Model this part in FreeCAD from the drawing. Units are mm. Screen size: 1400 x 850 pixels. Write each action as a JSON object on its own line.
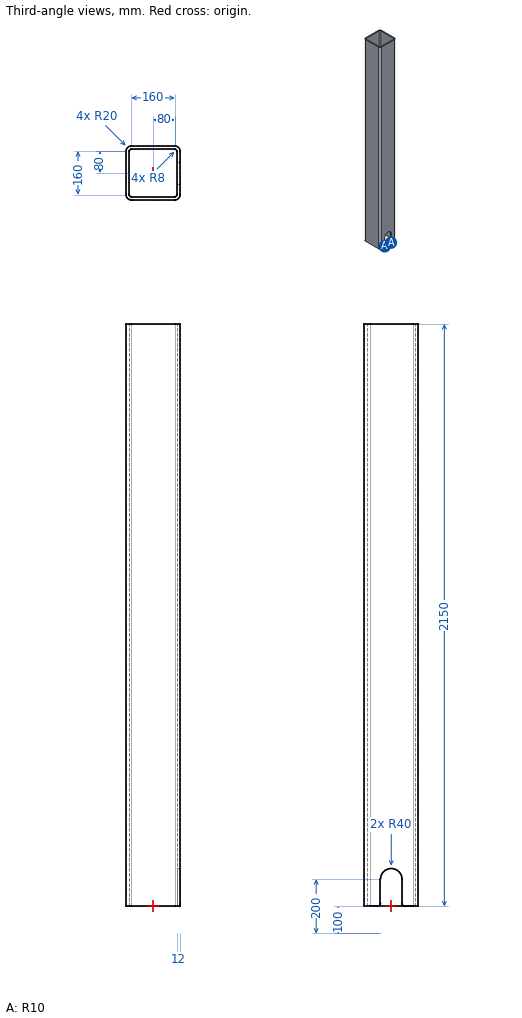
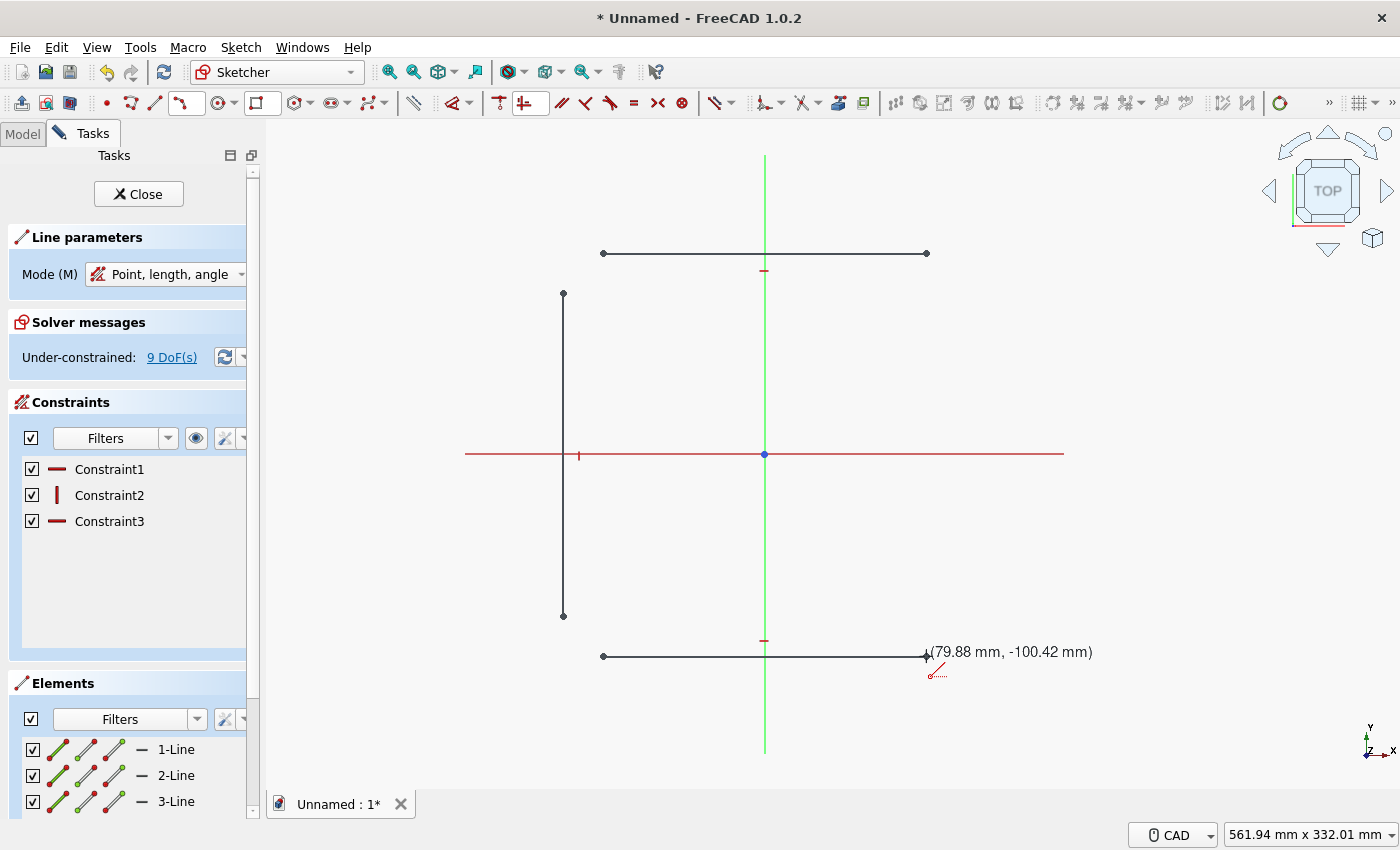
{"action": "left_click", "coordinate": [967, 616]}
{"action": "left_click", "coordinate": [967, 293]}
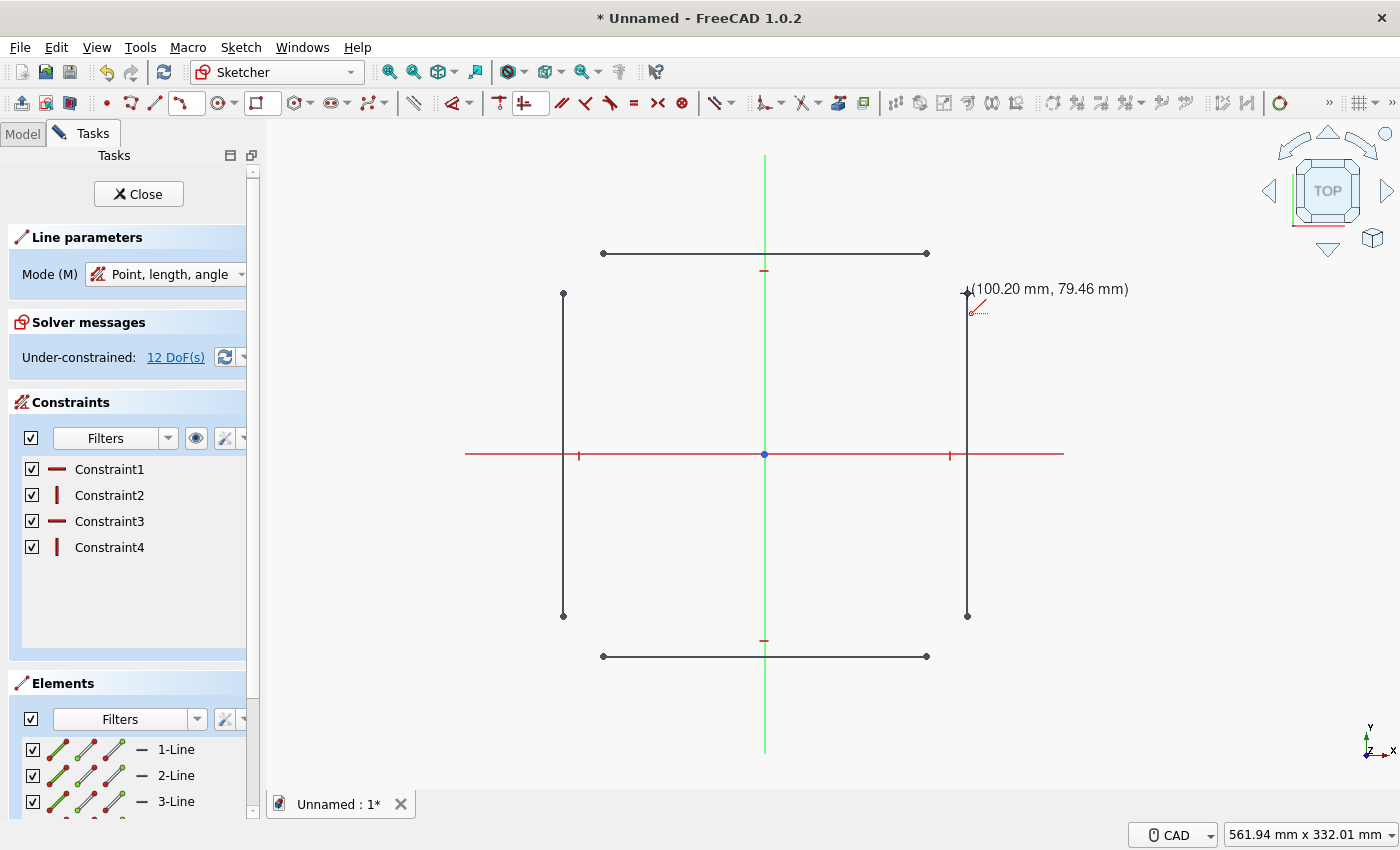
{"action": "left_click", "coordinate": [180, 104]}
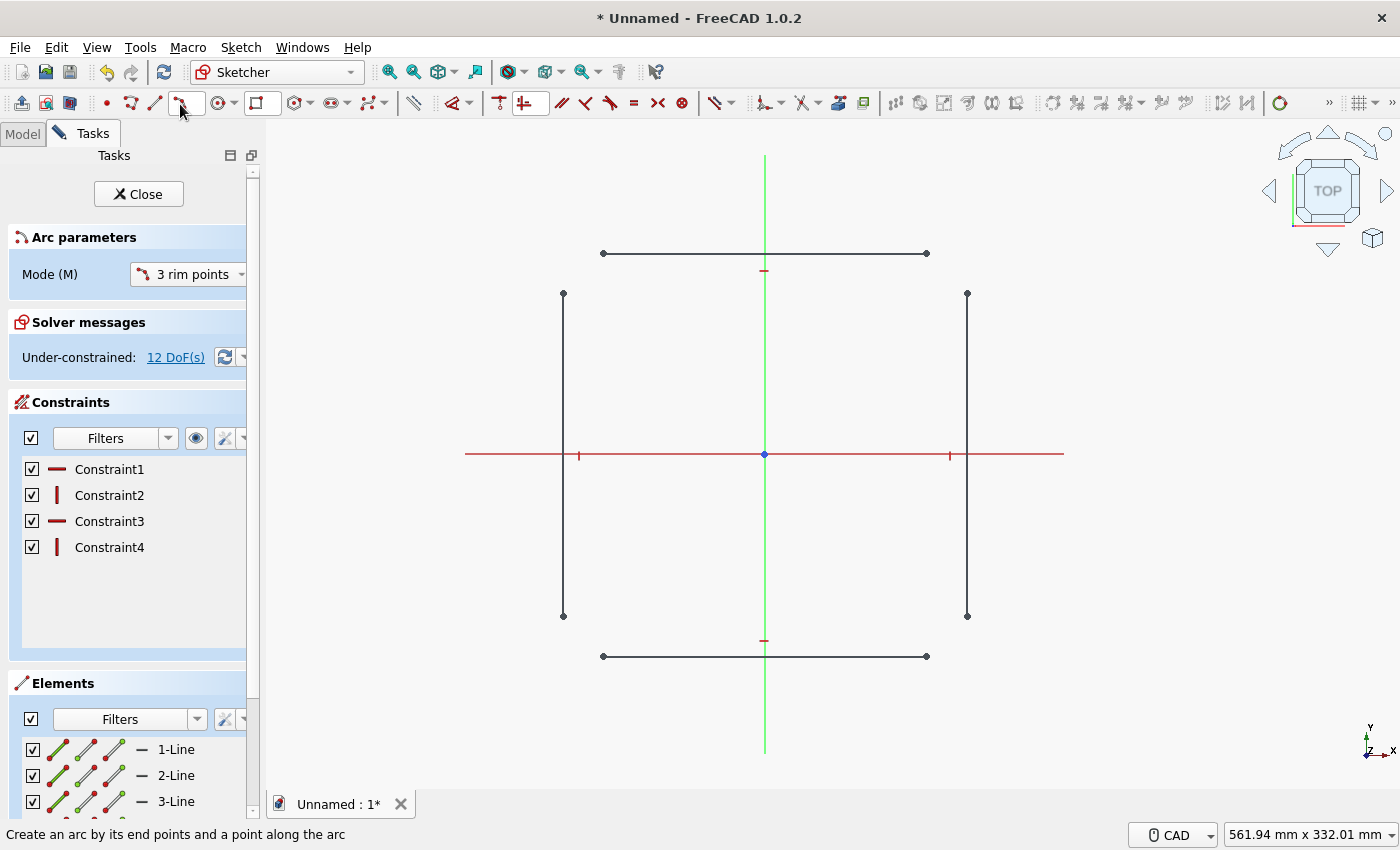
{"action": "left_click", "coordinate": [603, 254]}
{"action": "left_click", "coordinate": [563, 294]}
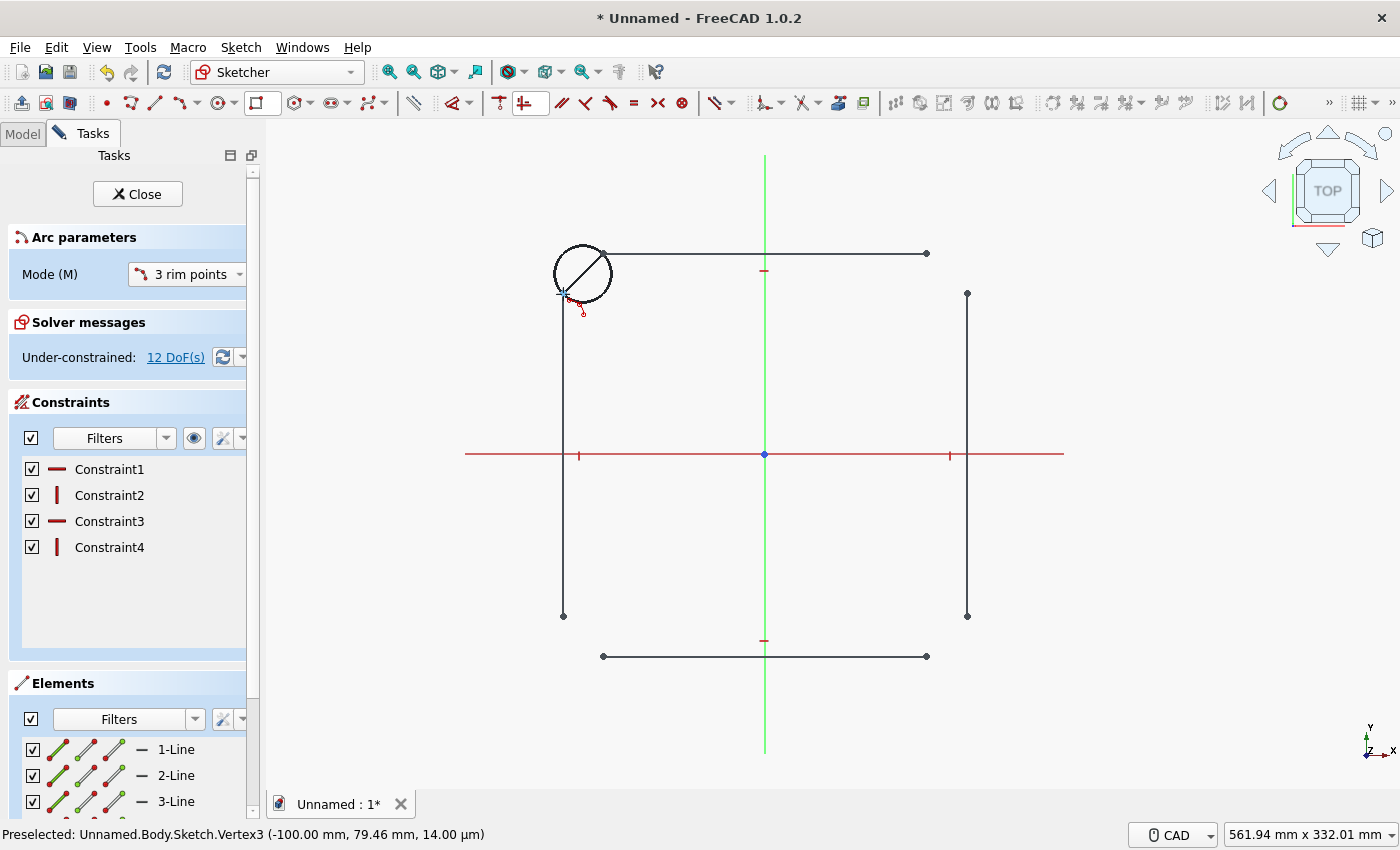
{"action": "scroll", "coordinate": [575, 264], "scroll_direction": "up", "scroll_amount": 2}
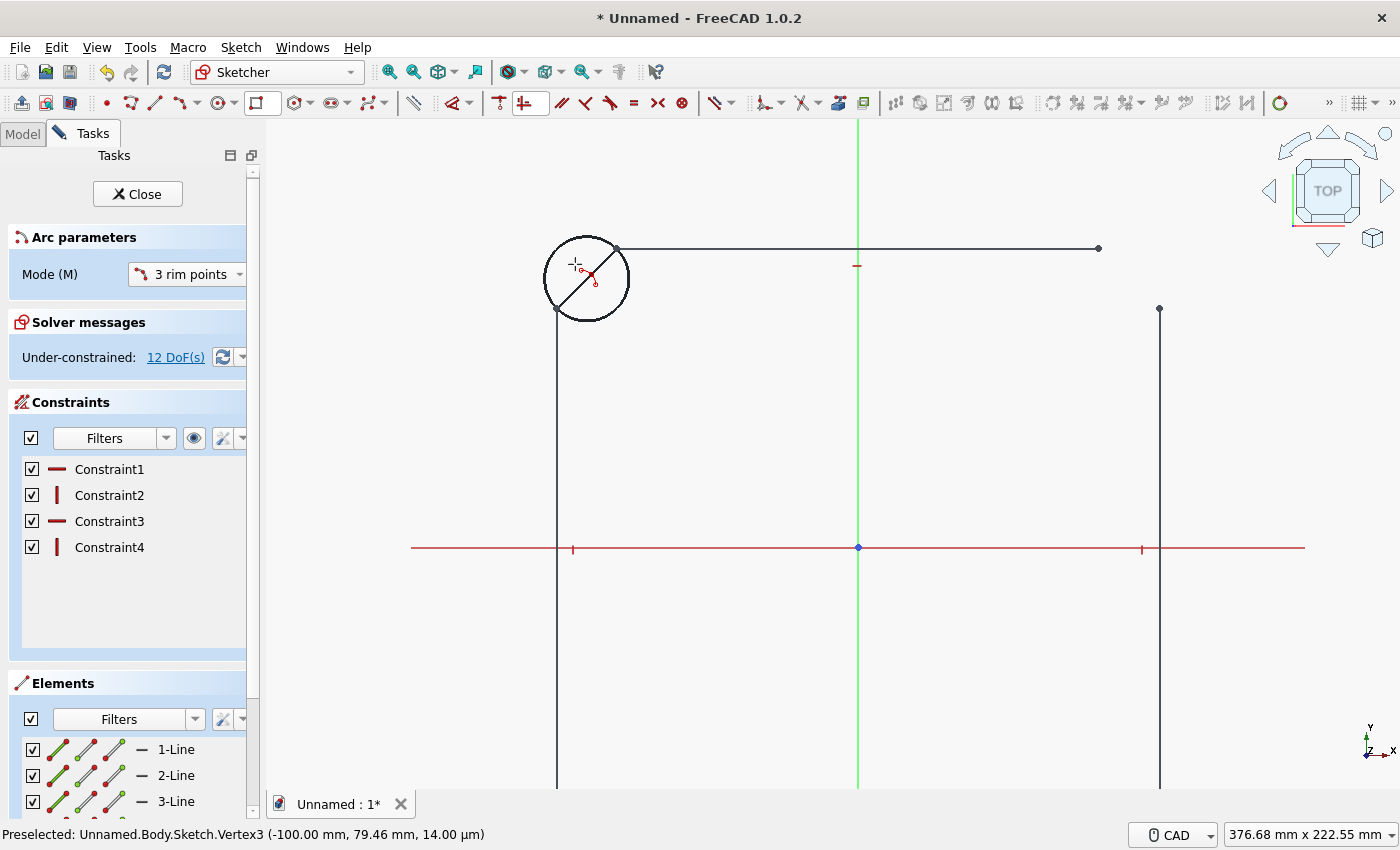
{"action": "left_click", "coordinate": [575, 264]}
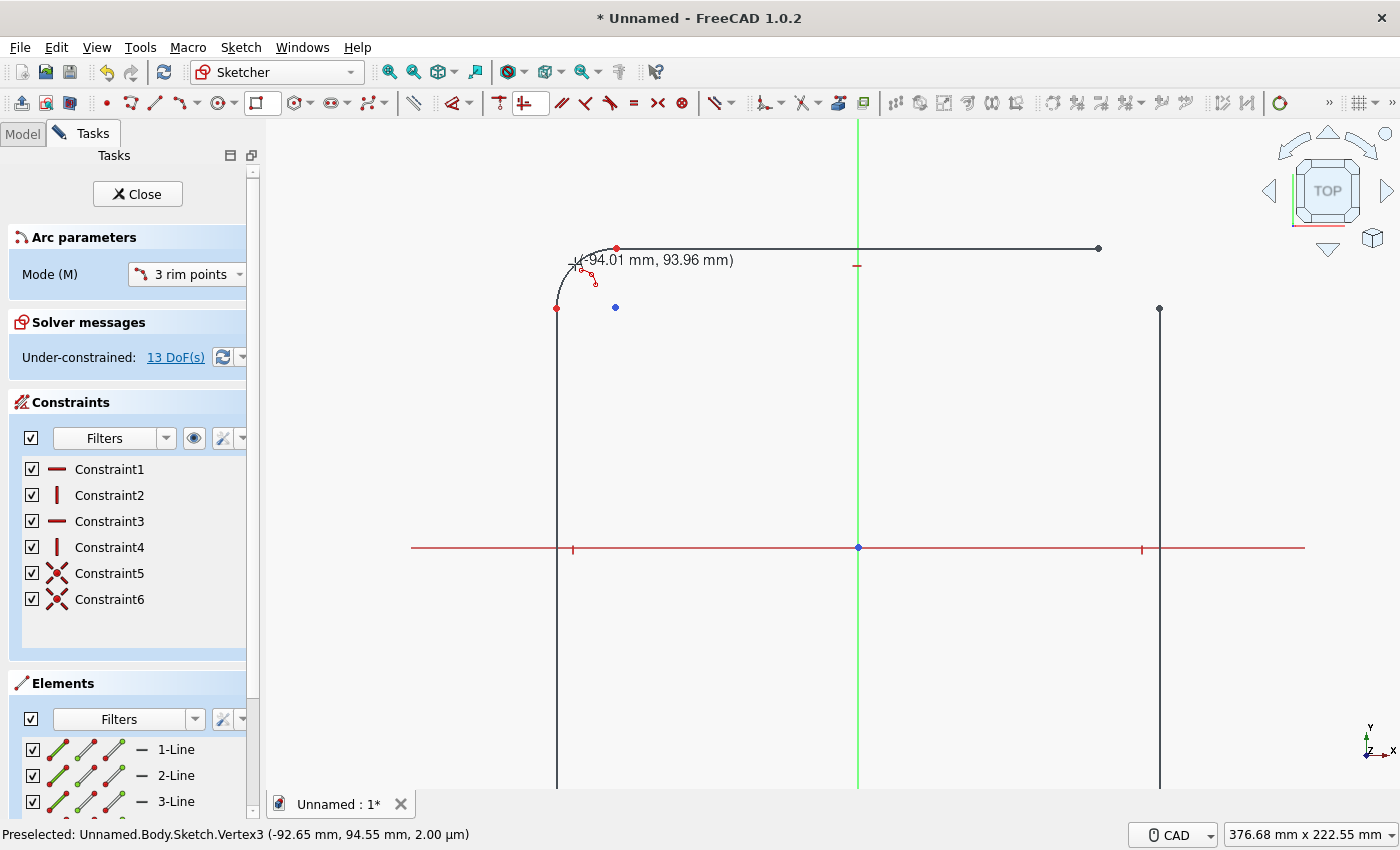
{"action": "scroll", "coordinate": [574, 263], "scroll_direction": "down", "scroll_amount": 2}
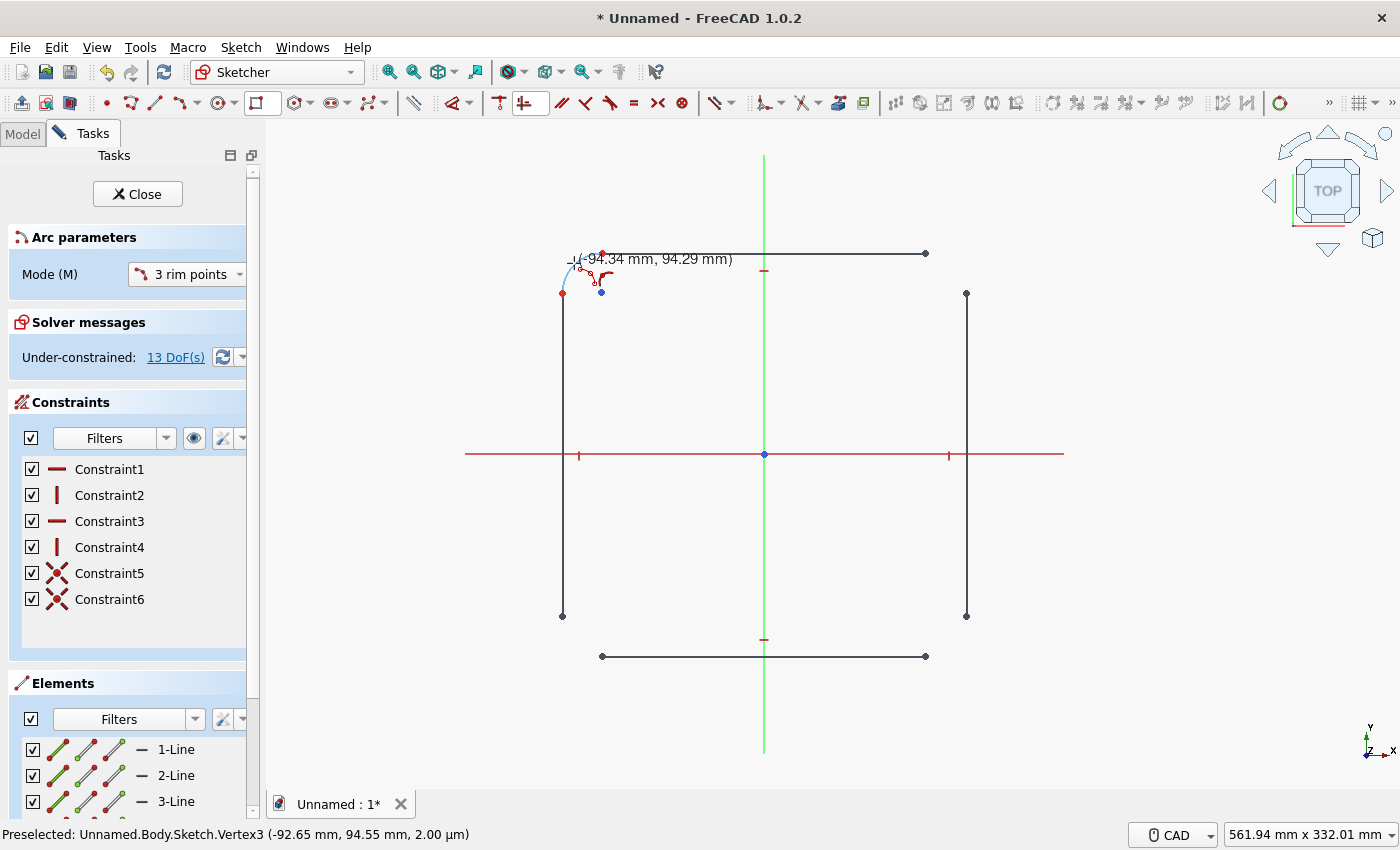
{"action": "left_click", "coordinate": [563, 617]}
{"action": "left_click", "coordinate": [603, 657]}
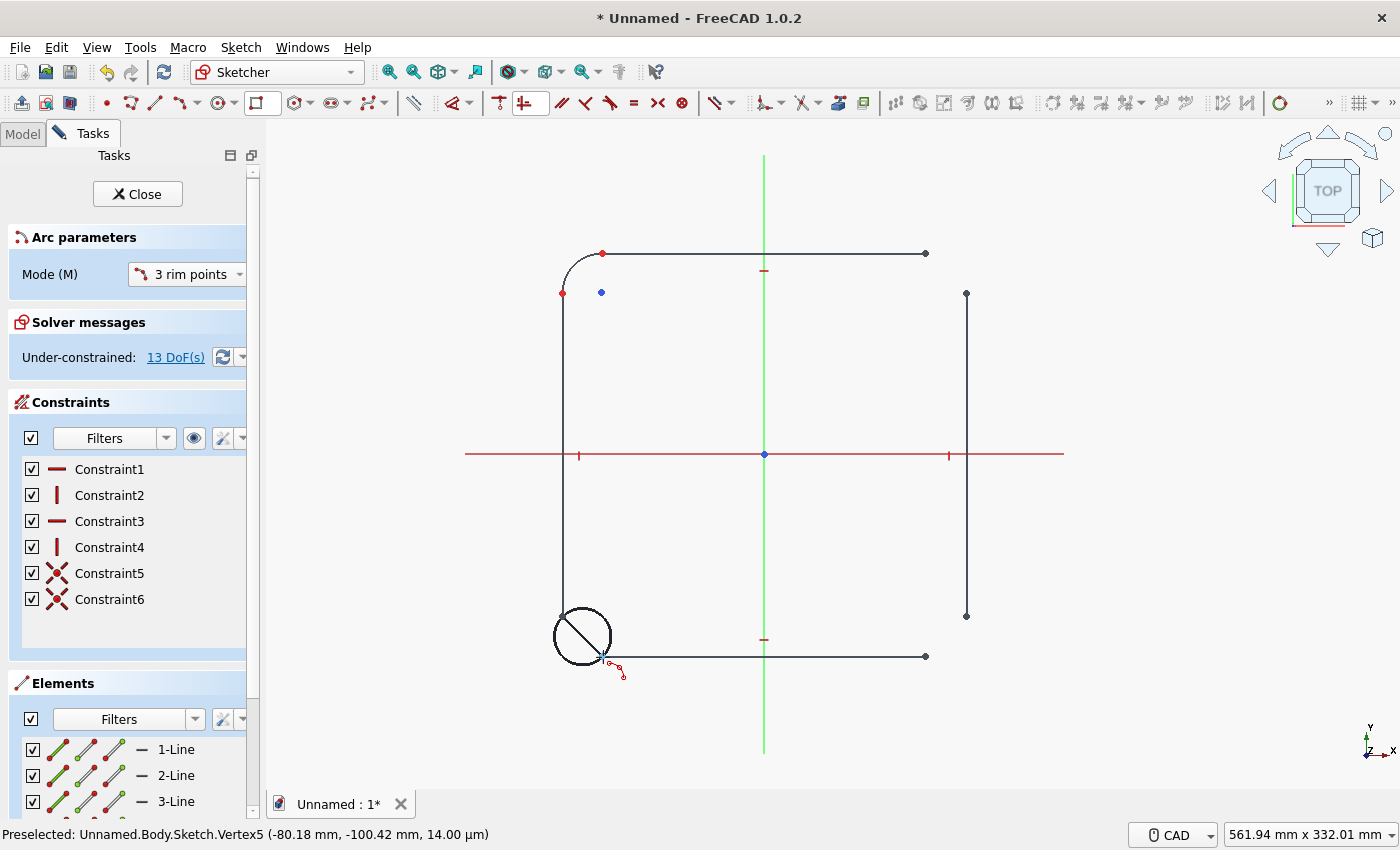
{"action": "scroll", "coordinate": [574, 644], "scroll_direction": "up", "scroll_amount": 2}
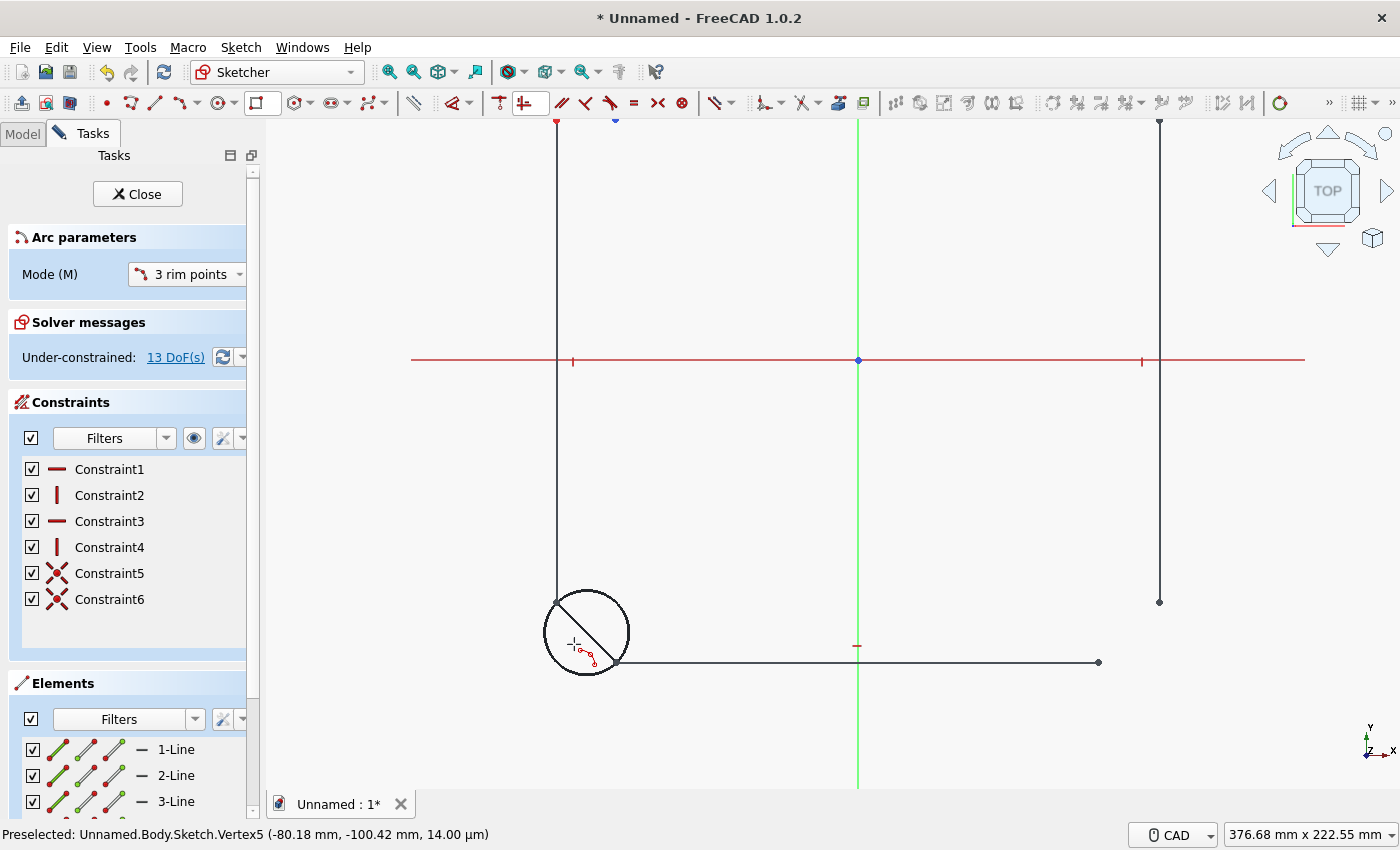
{"action": "left_click", "coordinate": [575, 644]}